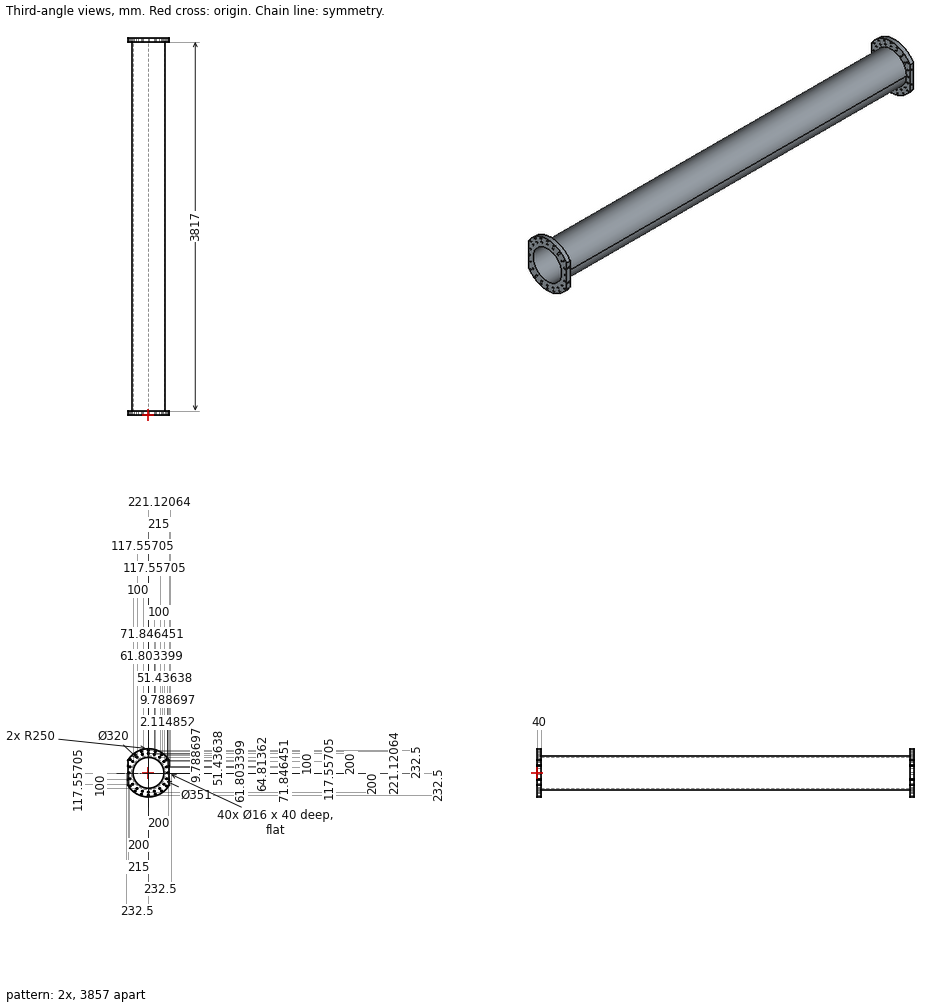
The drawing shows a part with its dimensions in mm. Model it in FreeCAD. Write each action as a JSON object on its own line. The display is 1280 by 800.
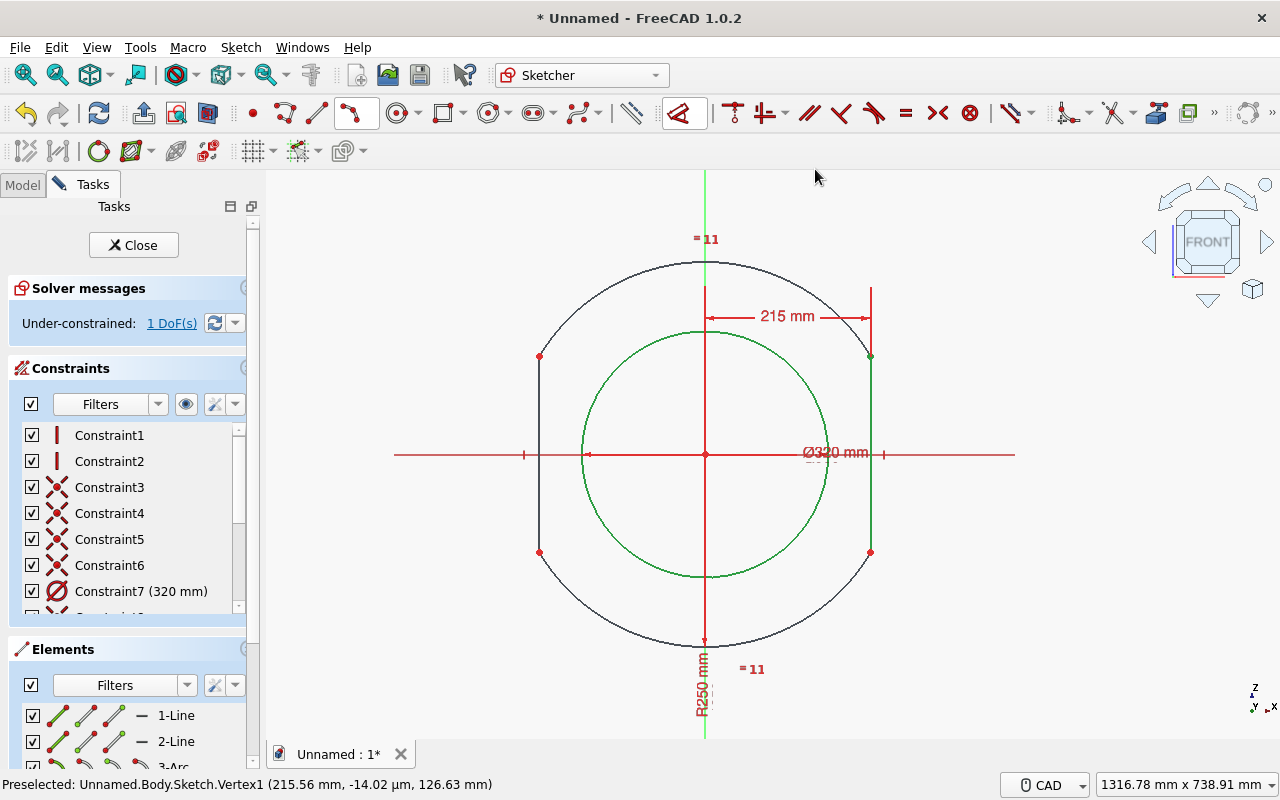
{"action": "left_click", "coordinate": [539, 552]}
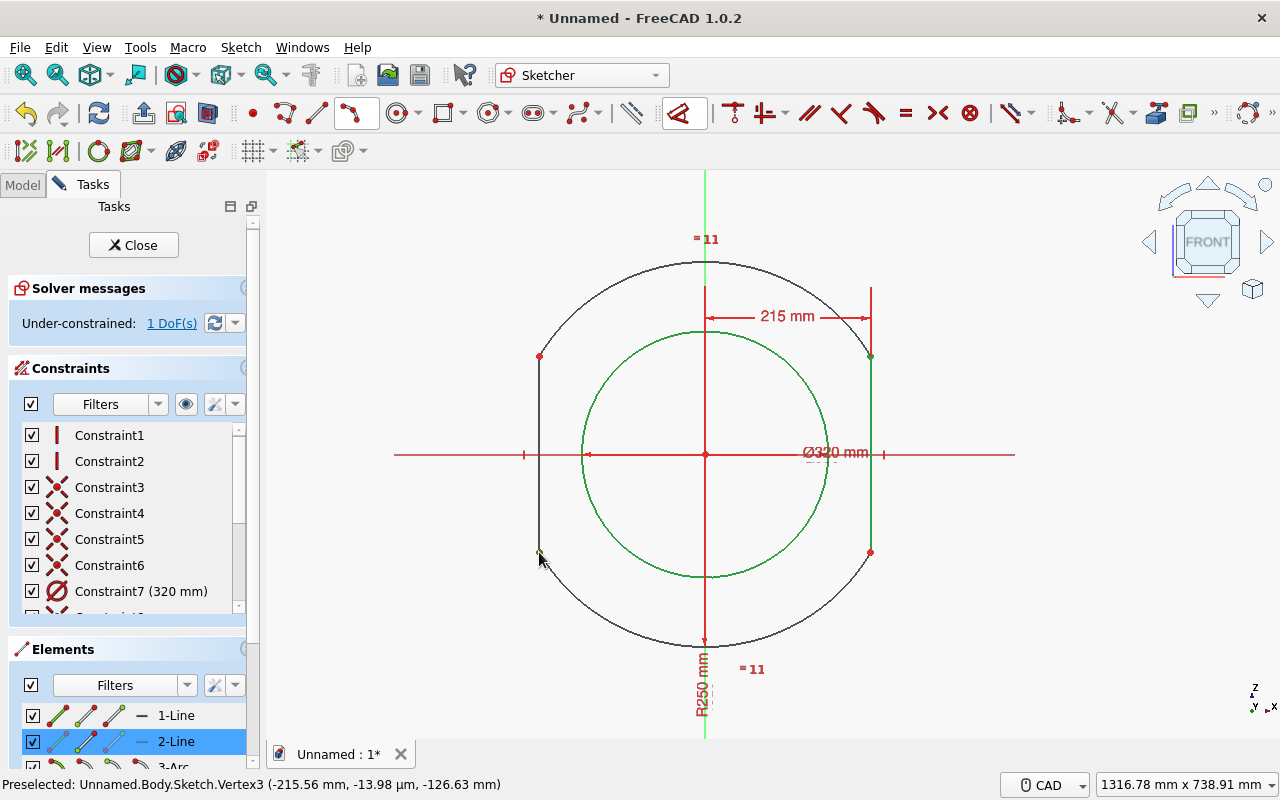
{"action": "left_click", "coordinate": [702, 114]}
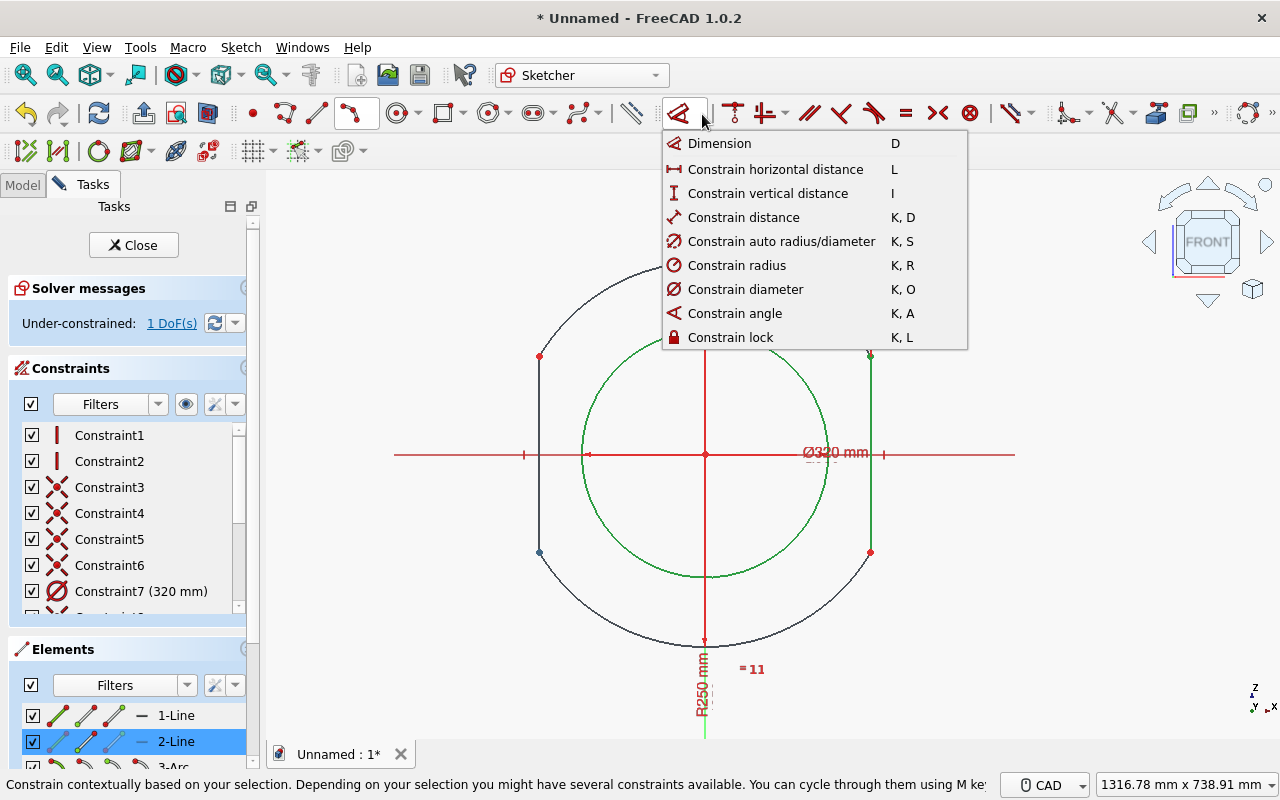
{"action": "left_click", "coordinate": [815, 169]}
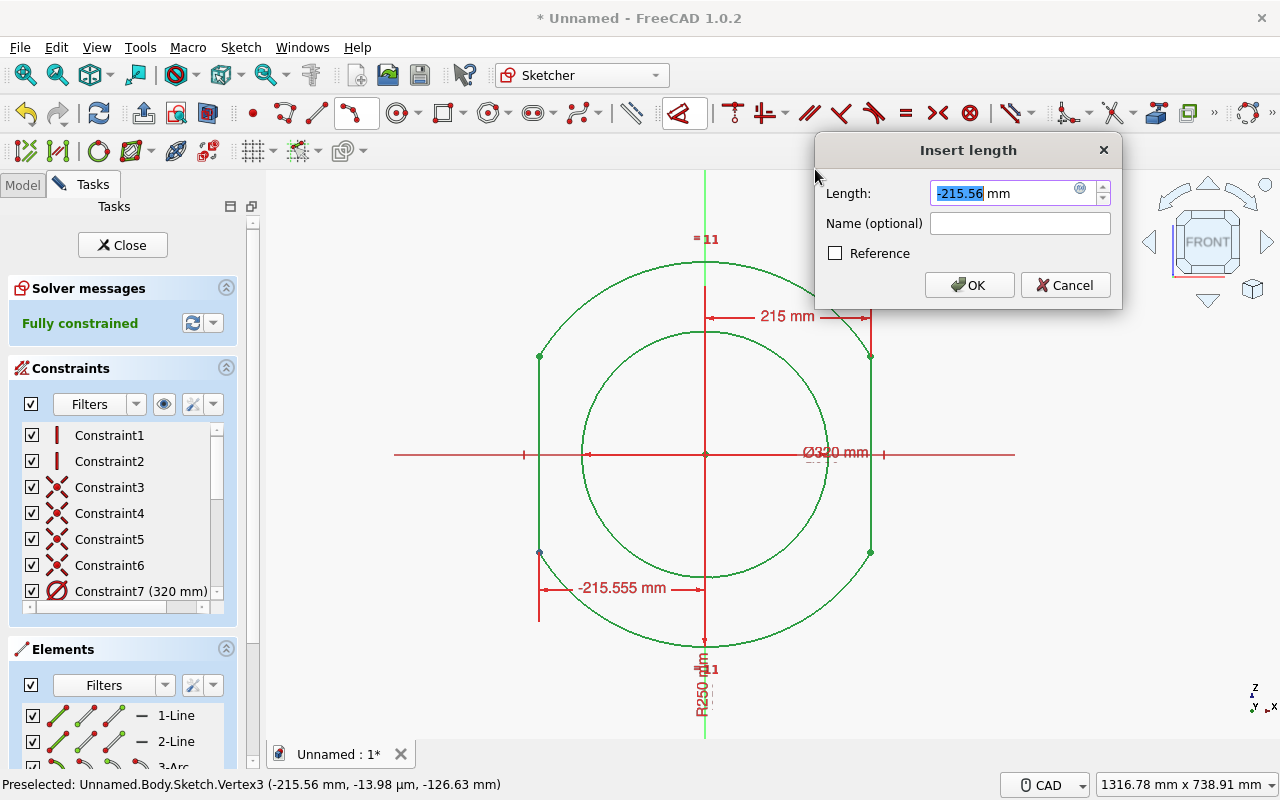
{"action": "type", "text": "-215"}
{"action": "key", "text": "Return"}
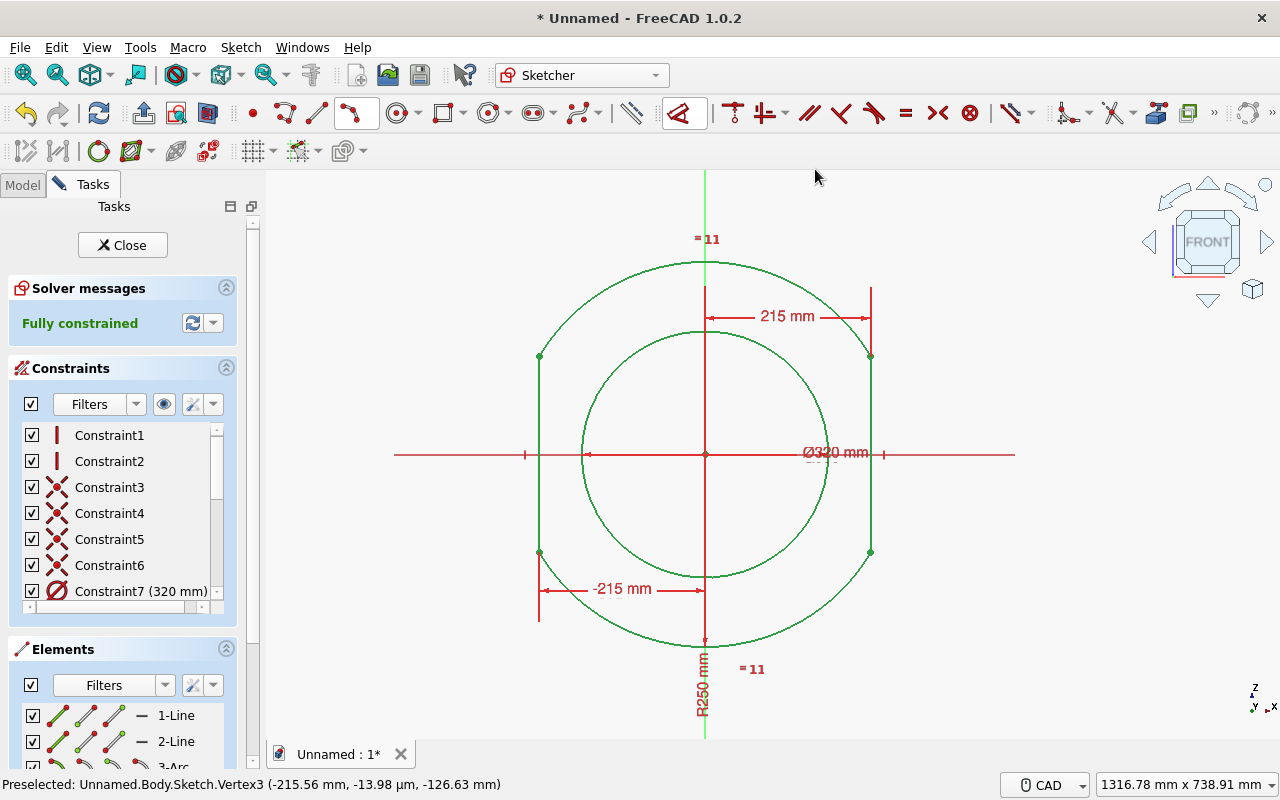
{"action": "left_click", "coordinate": [123, 245]}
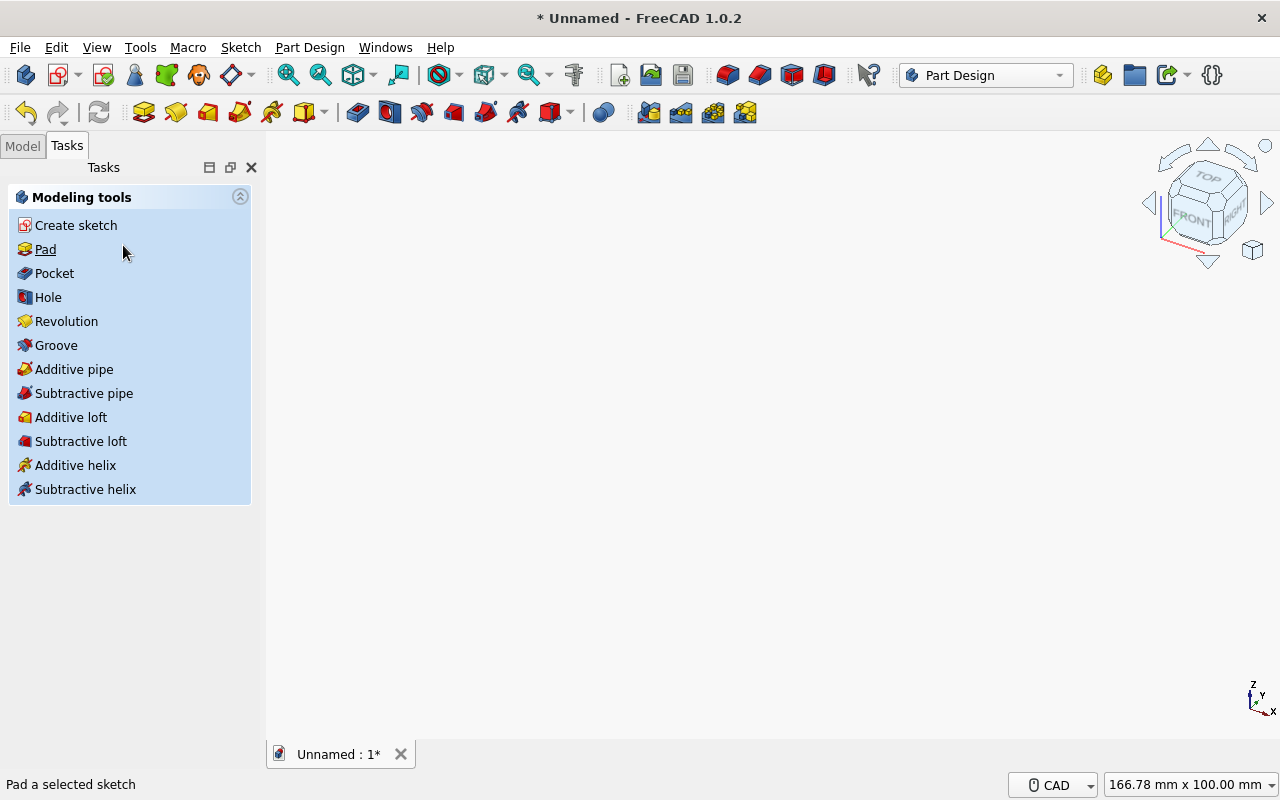
{"action": "left_click", "coordinate": [144, 112]}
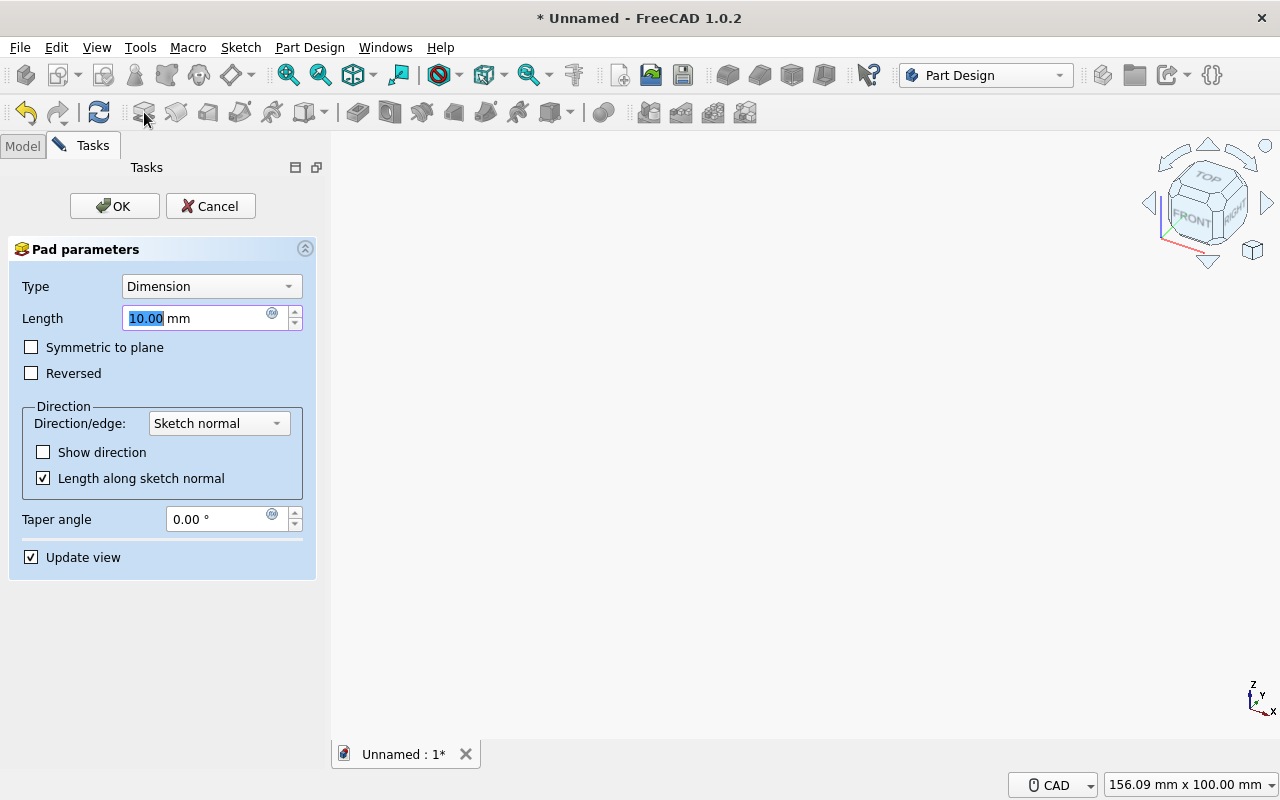
{"action": "type", "text": "40"}
{"action": "key", "text": "Tab"}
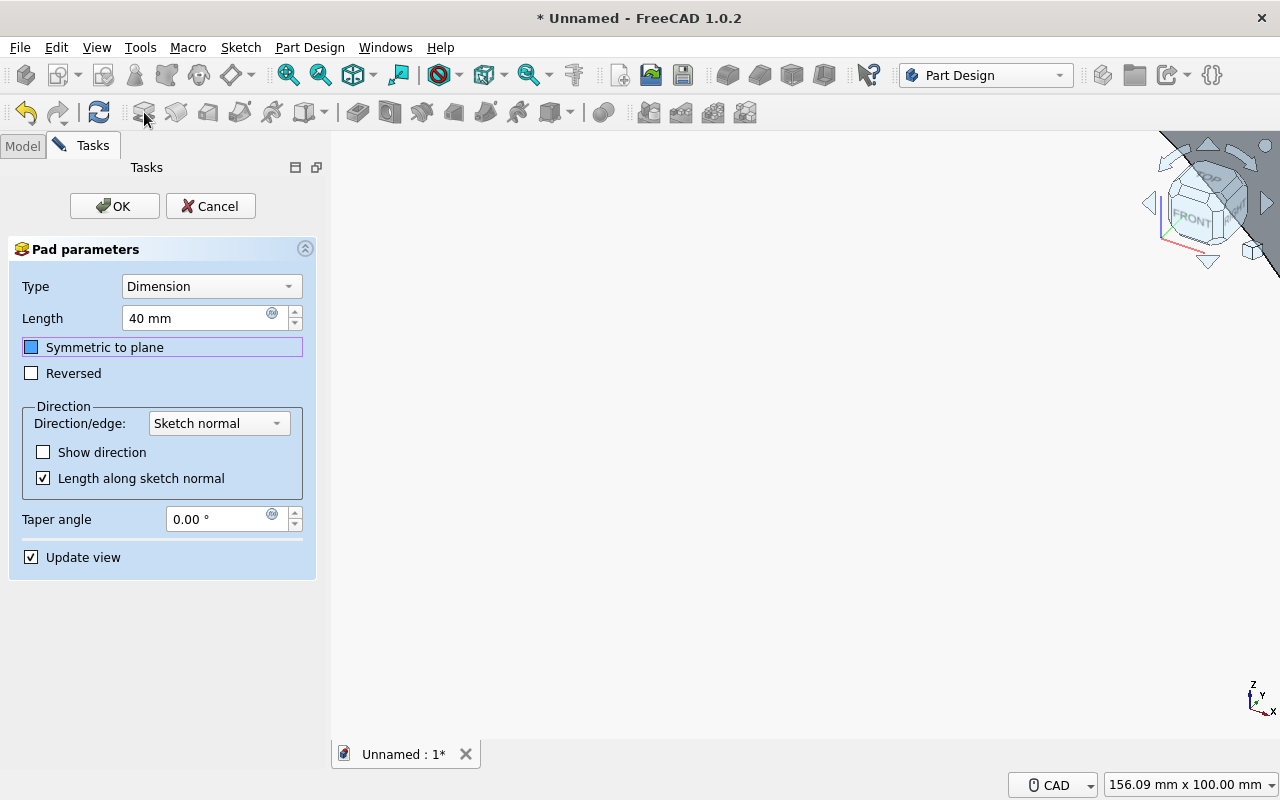
{"action": "left_click", "coordinate": [30, 373]}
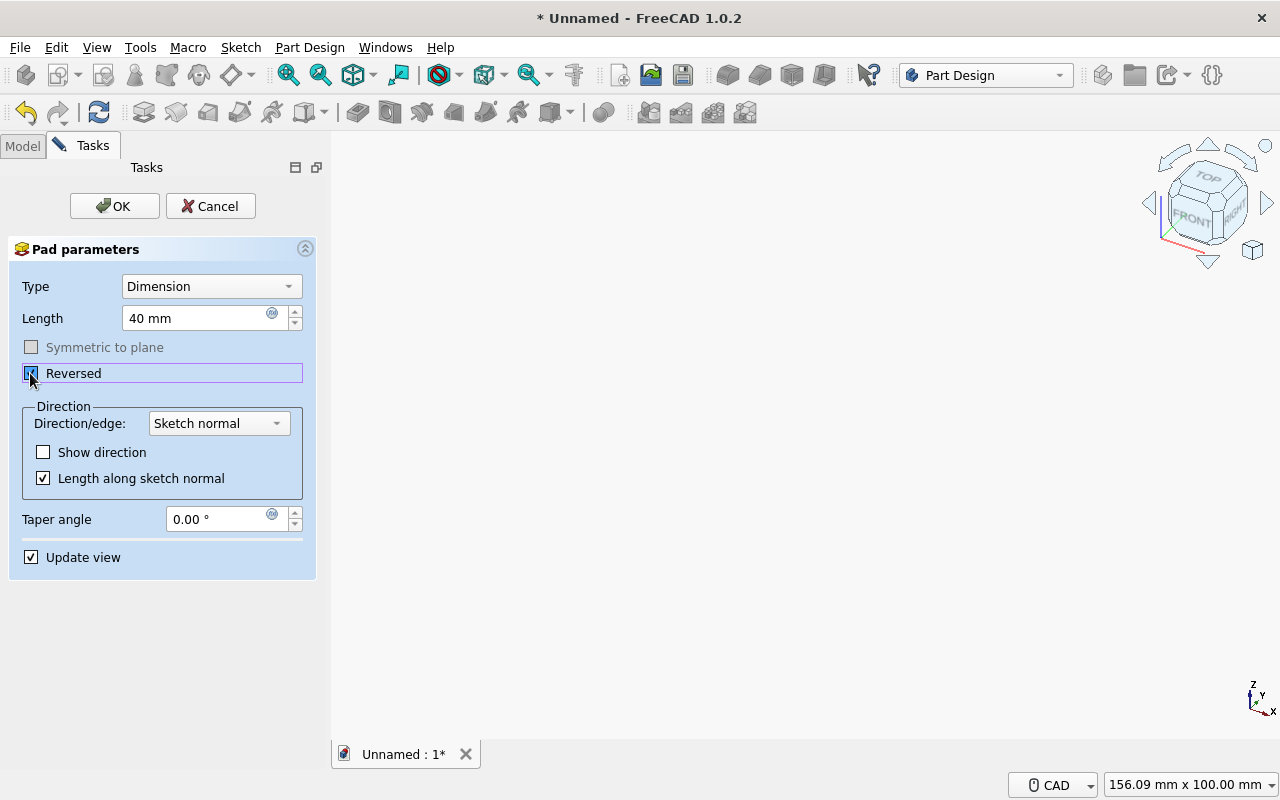
{"action": "left_click", "coordinate": [115, 206]}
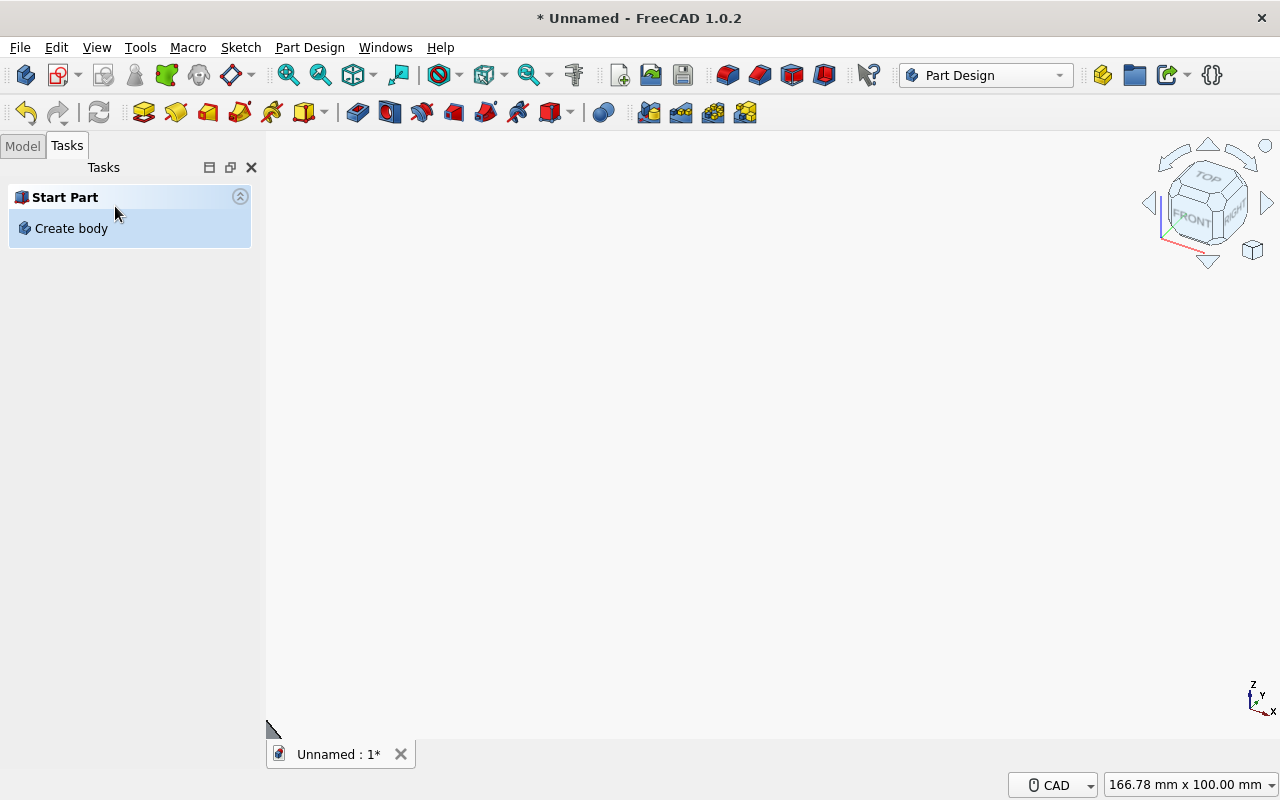
{"action": "left_click", "coordinate": [290, 76]}